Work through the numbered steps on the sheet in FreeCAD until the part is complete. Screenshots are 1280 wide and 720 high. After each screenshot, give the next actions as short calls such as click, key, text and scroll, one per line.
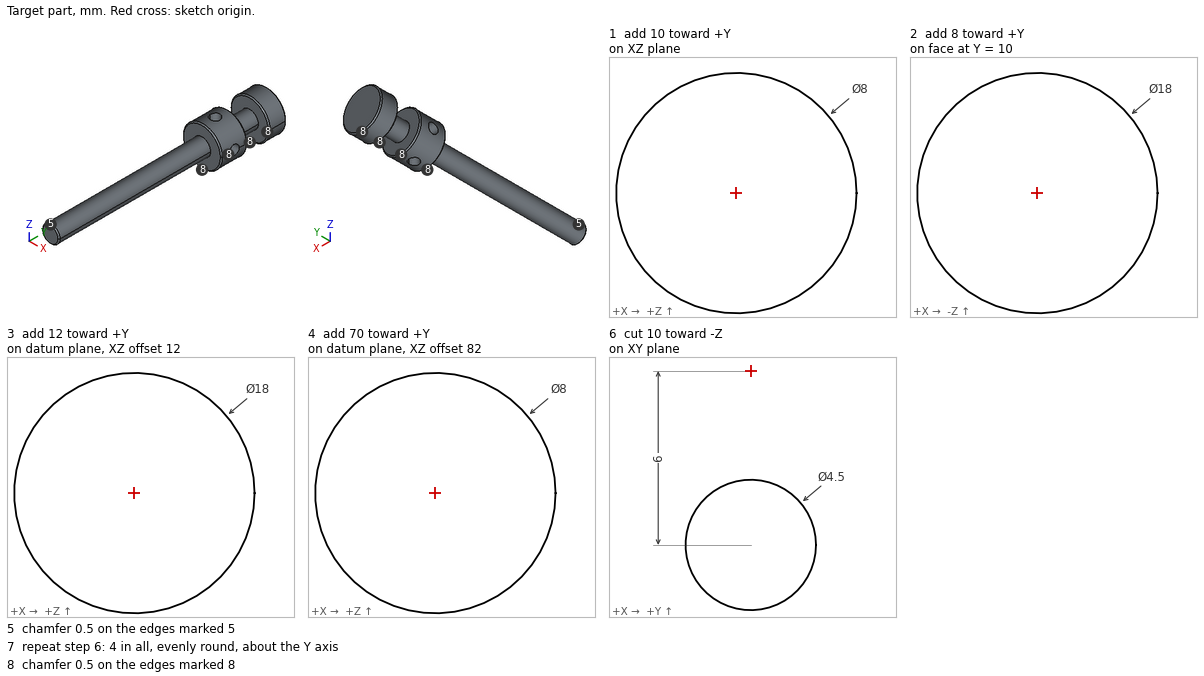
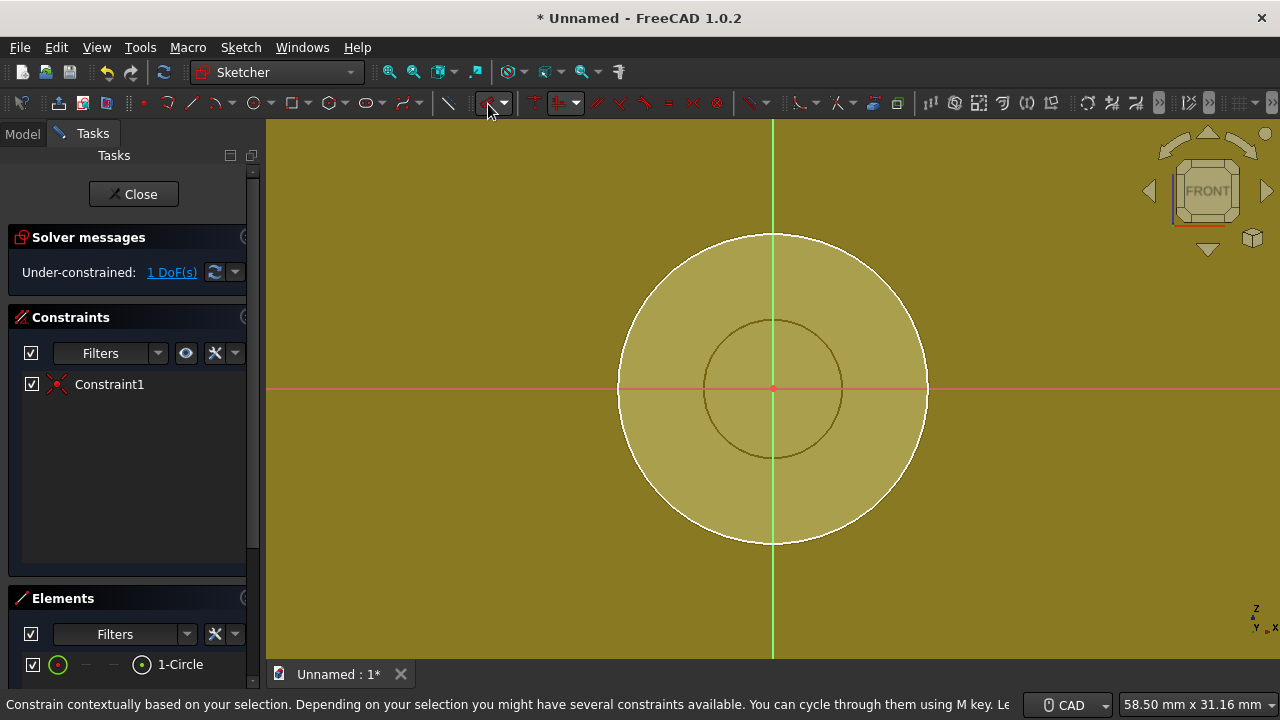
click(882, 279)
click(905, 256)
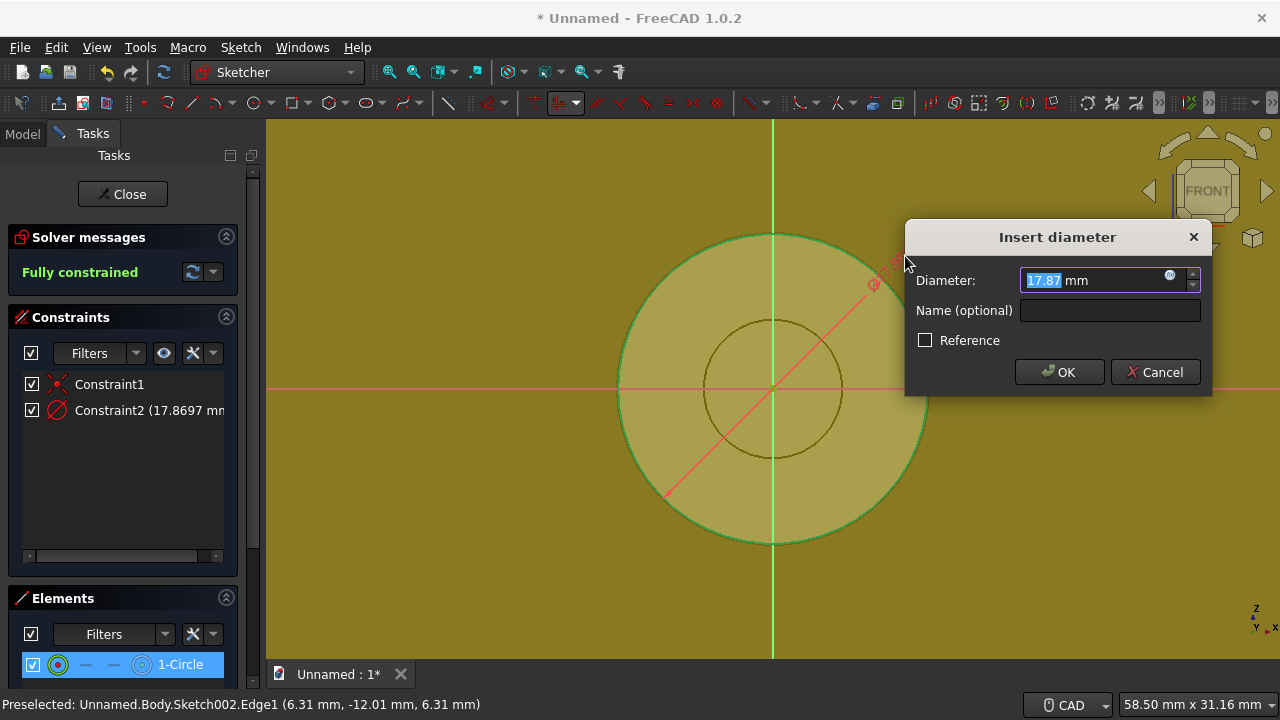
text(18)
key(Return)
key(Escape)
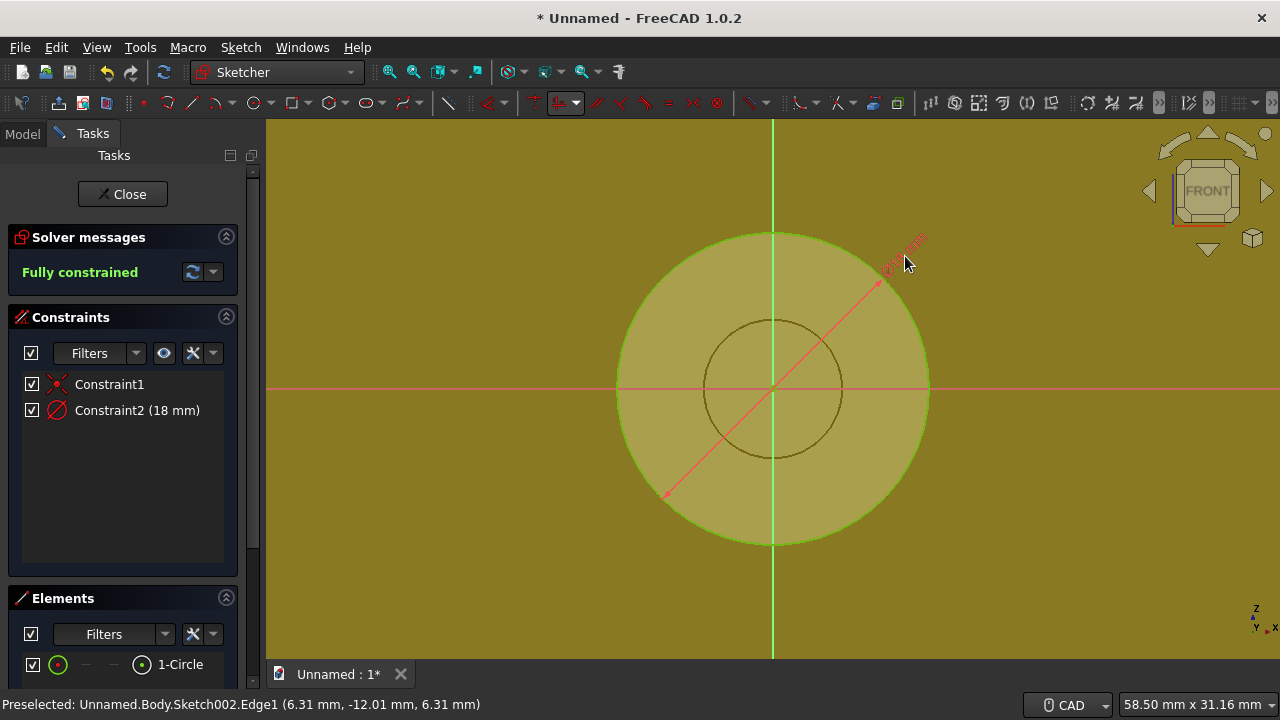
click(123, 194)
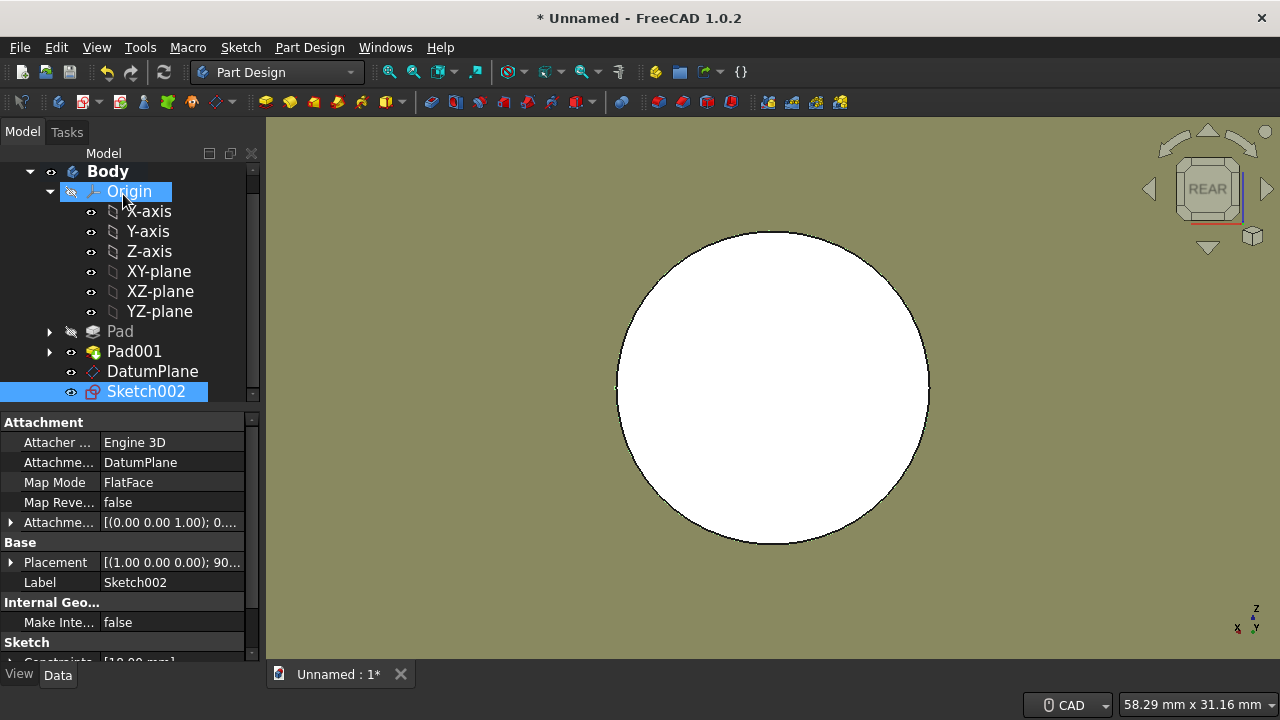
click(266, 102)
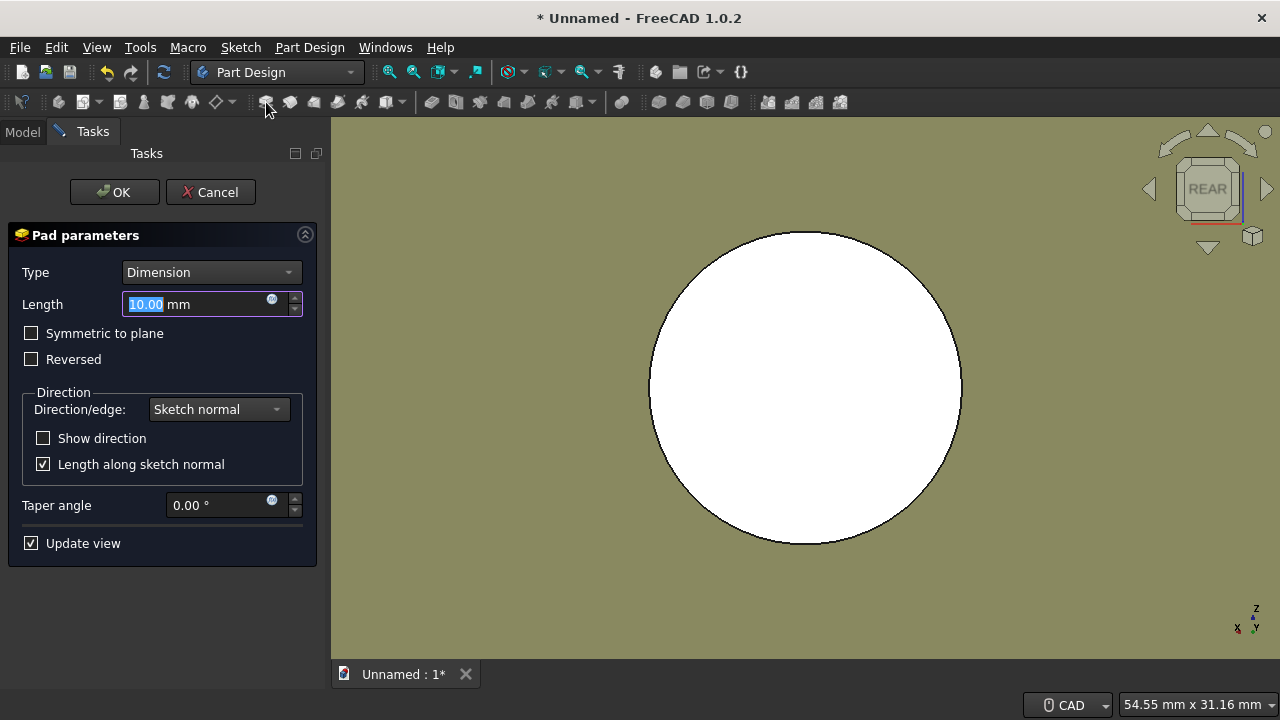
text(12)
key(Tab)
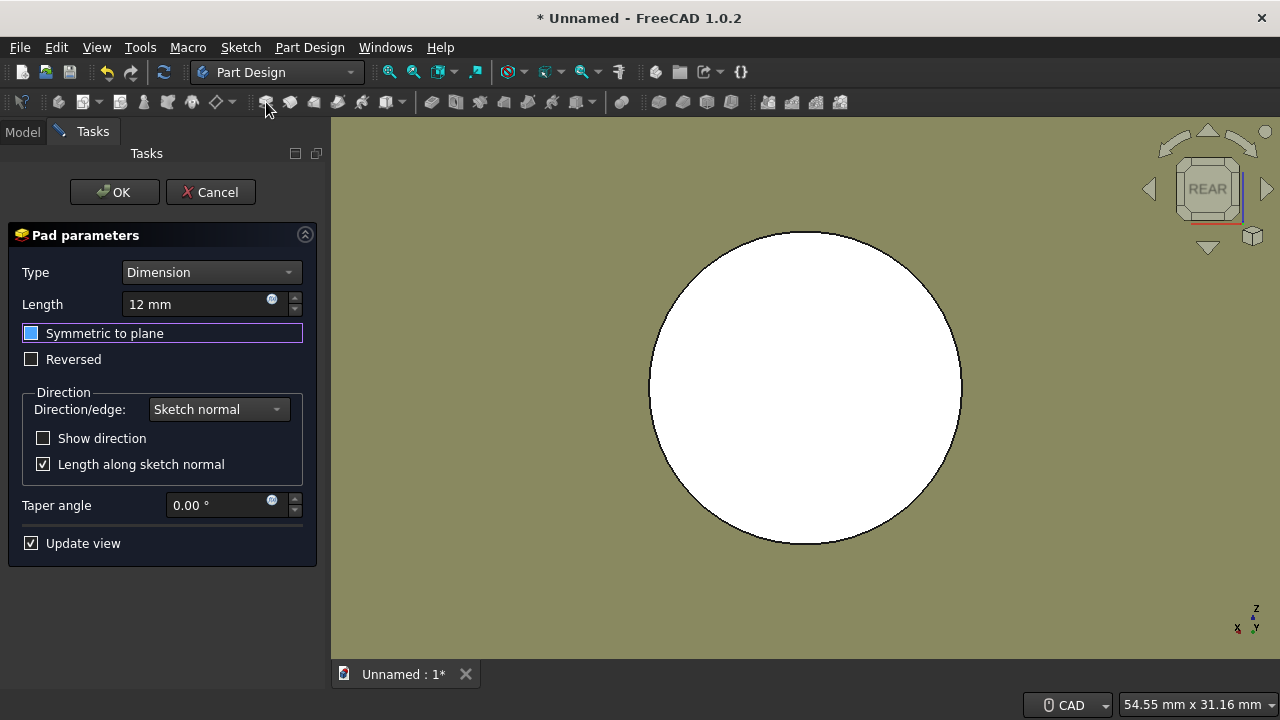
click(30, 359)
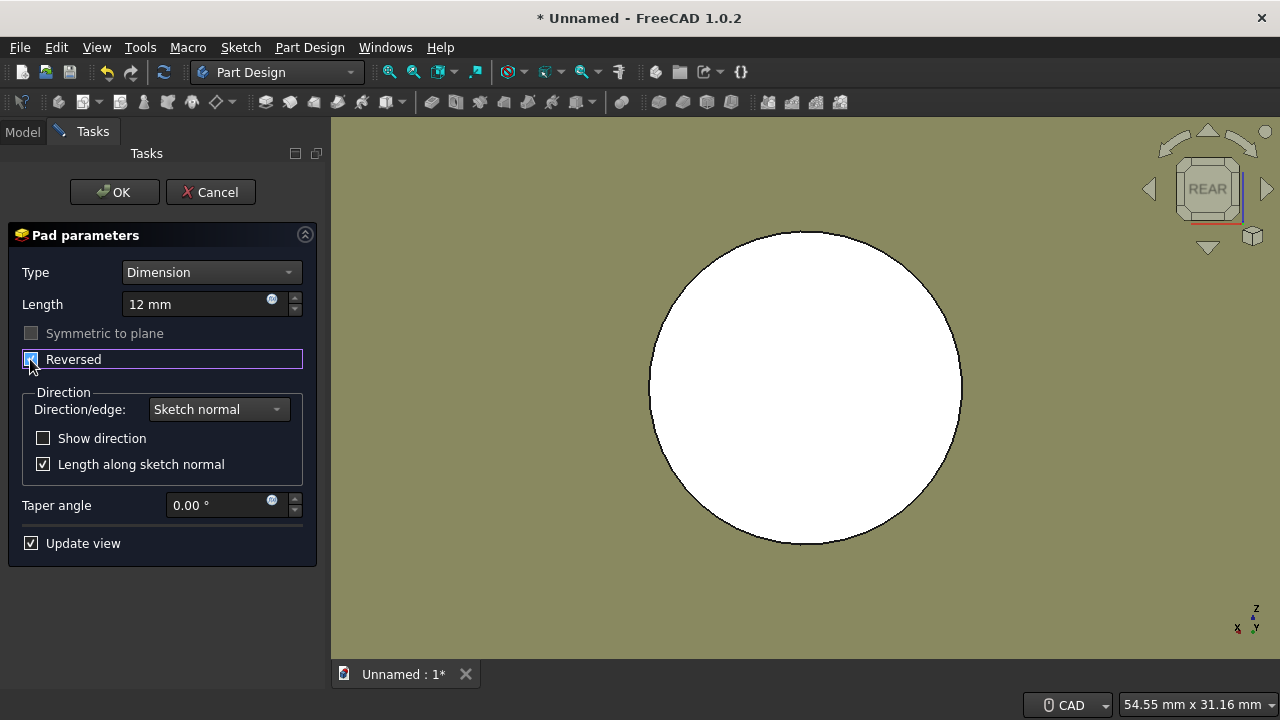
click(115, 192)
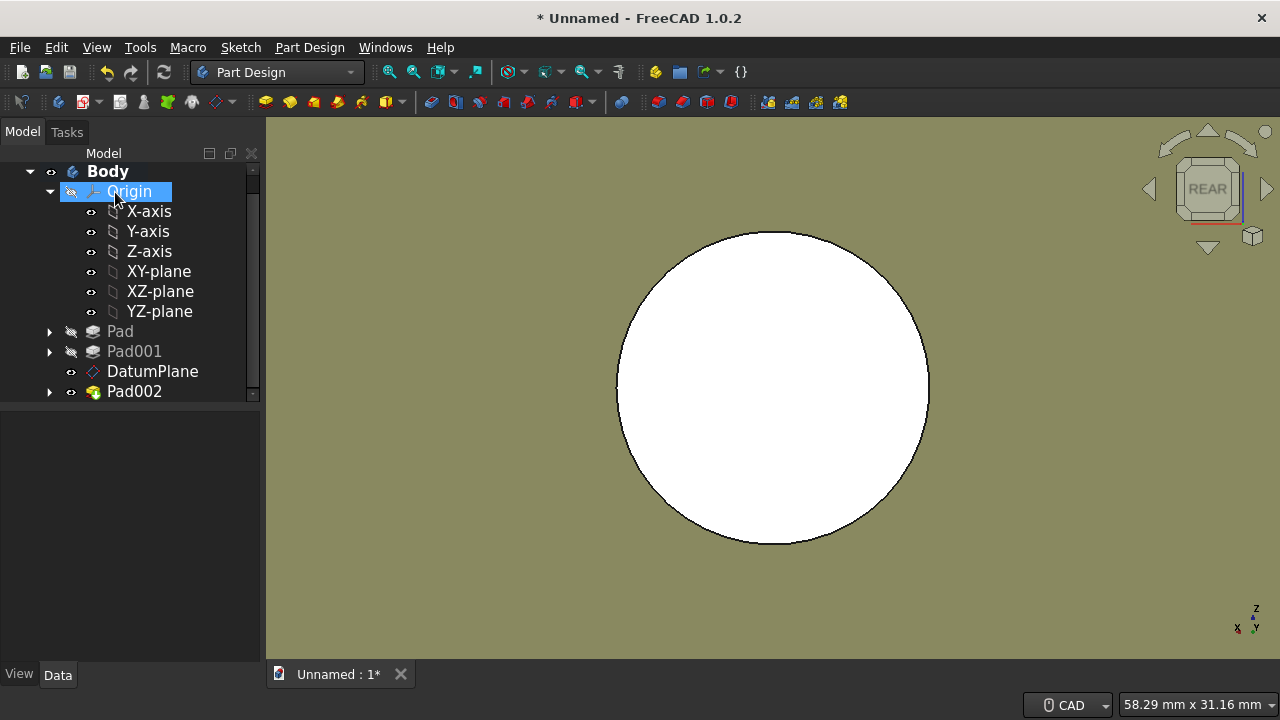
click(116, 372)
key(space)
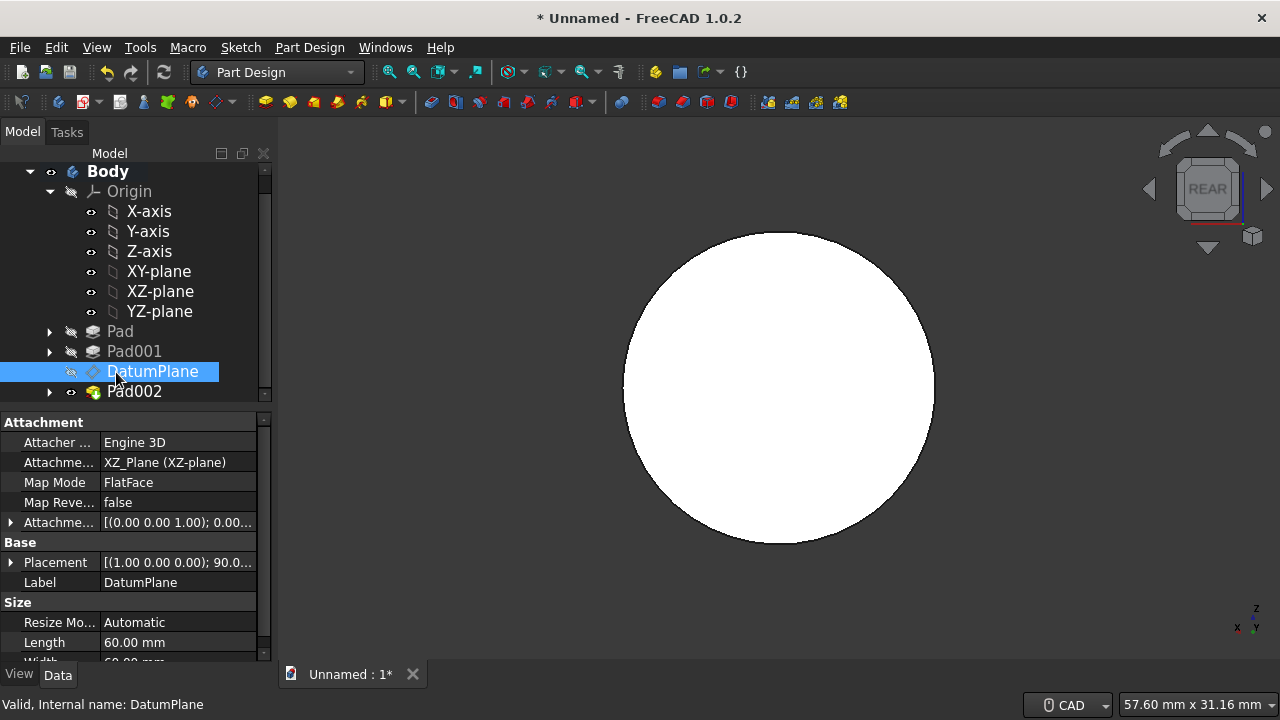
click(136, 292)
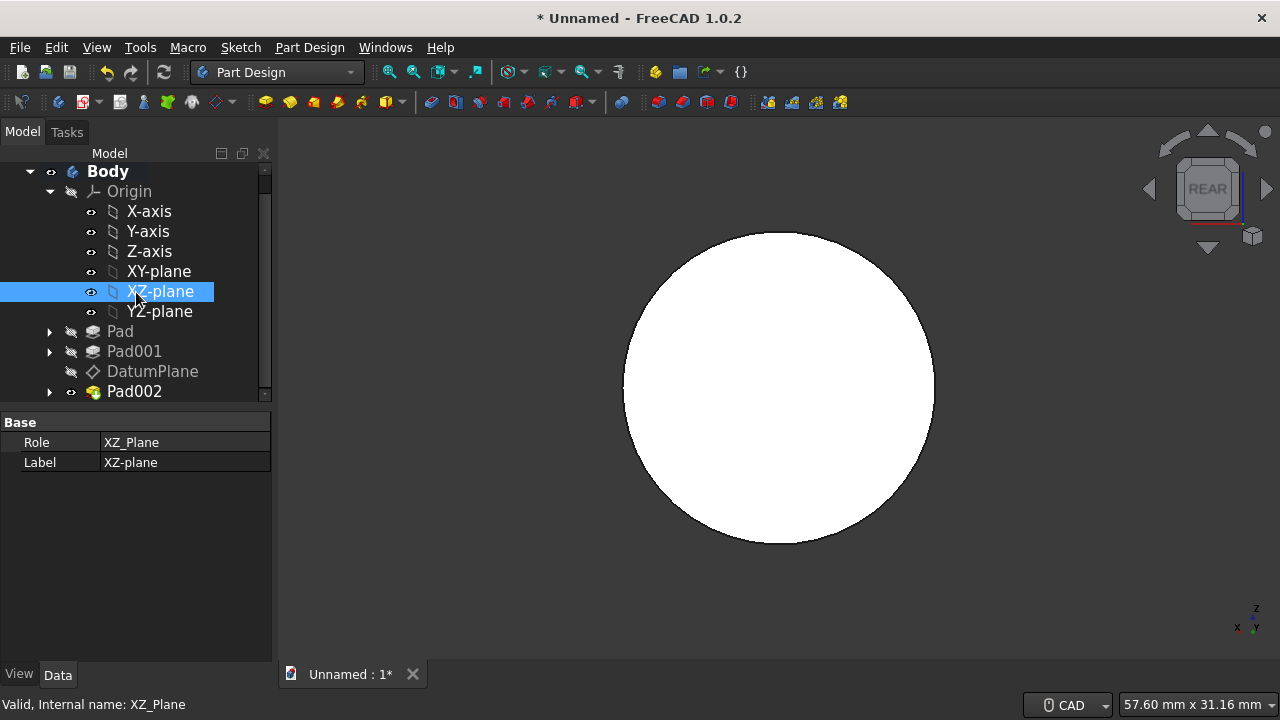
click(216, 102)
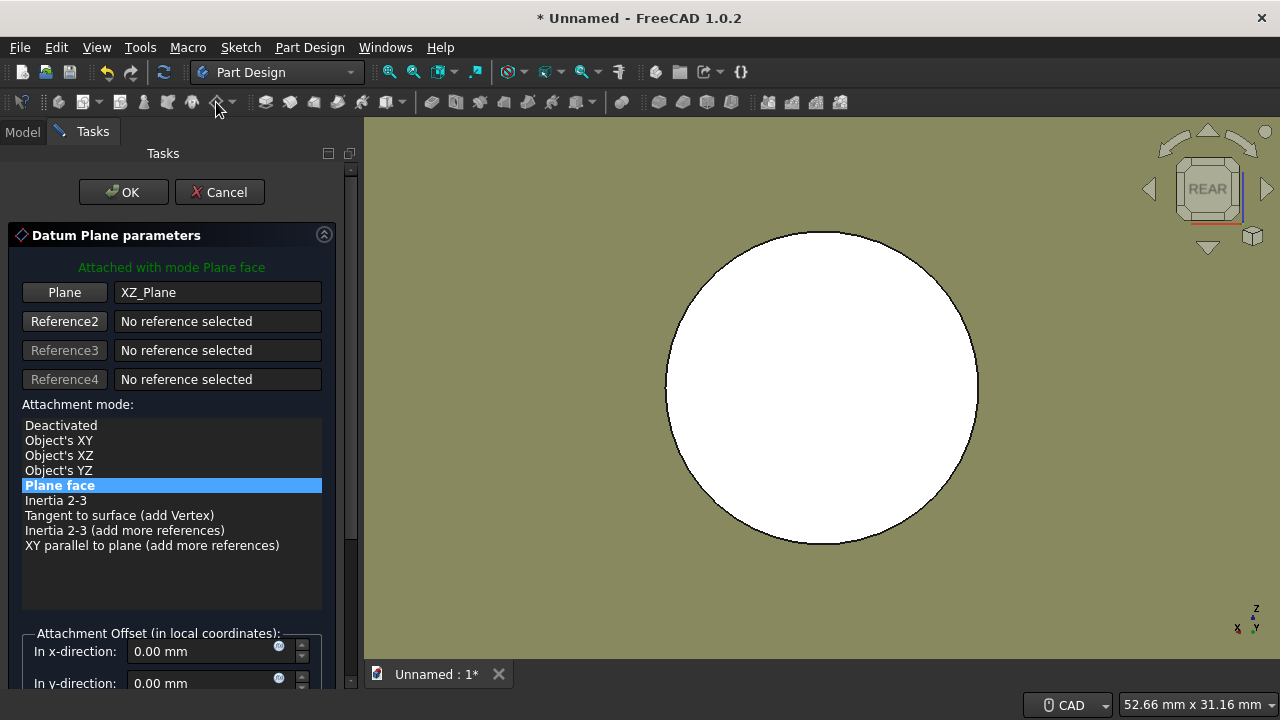
scroll(351, 426, down, 2)